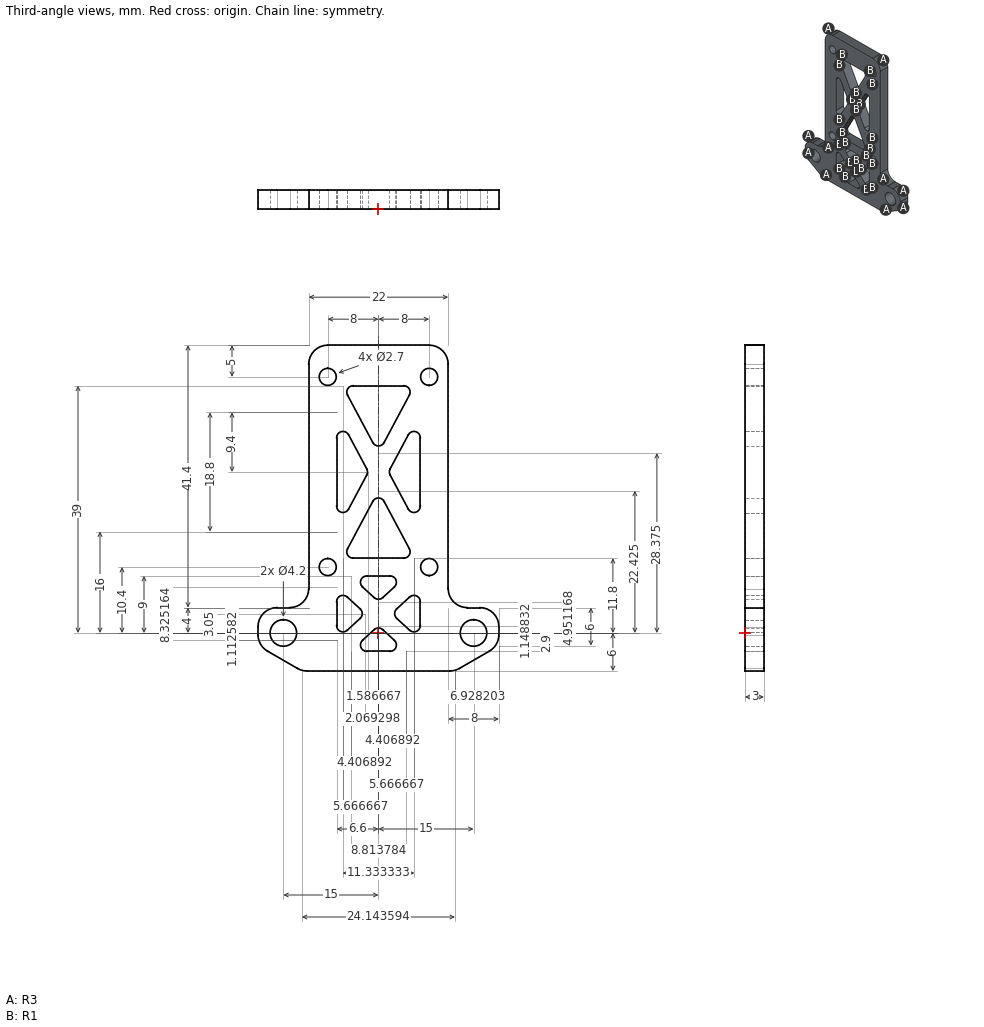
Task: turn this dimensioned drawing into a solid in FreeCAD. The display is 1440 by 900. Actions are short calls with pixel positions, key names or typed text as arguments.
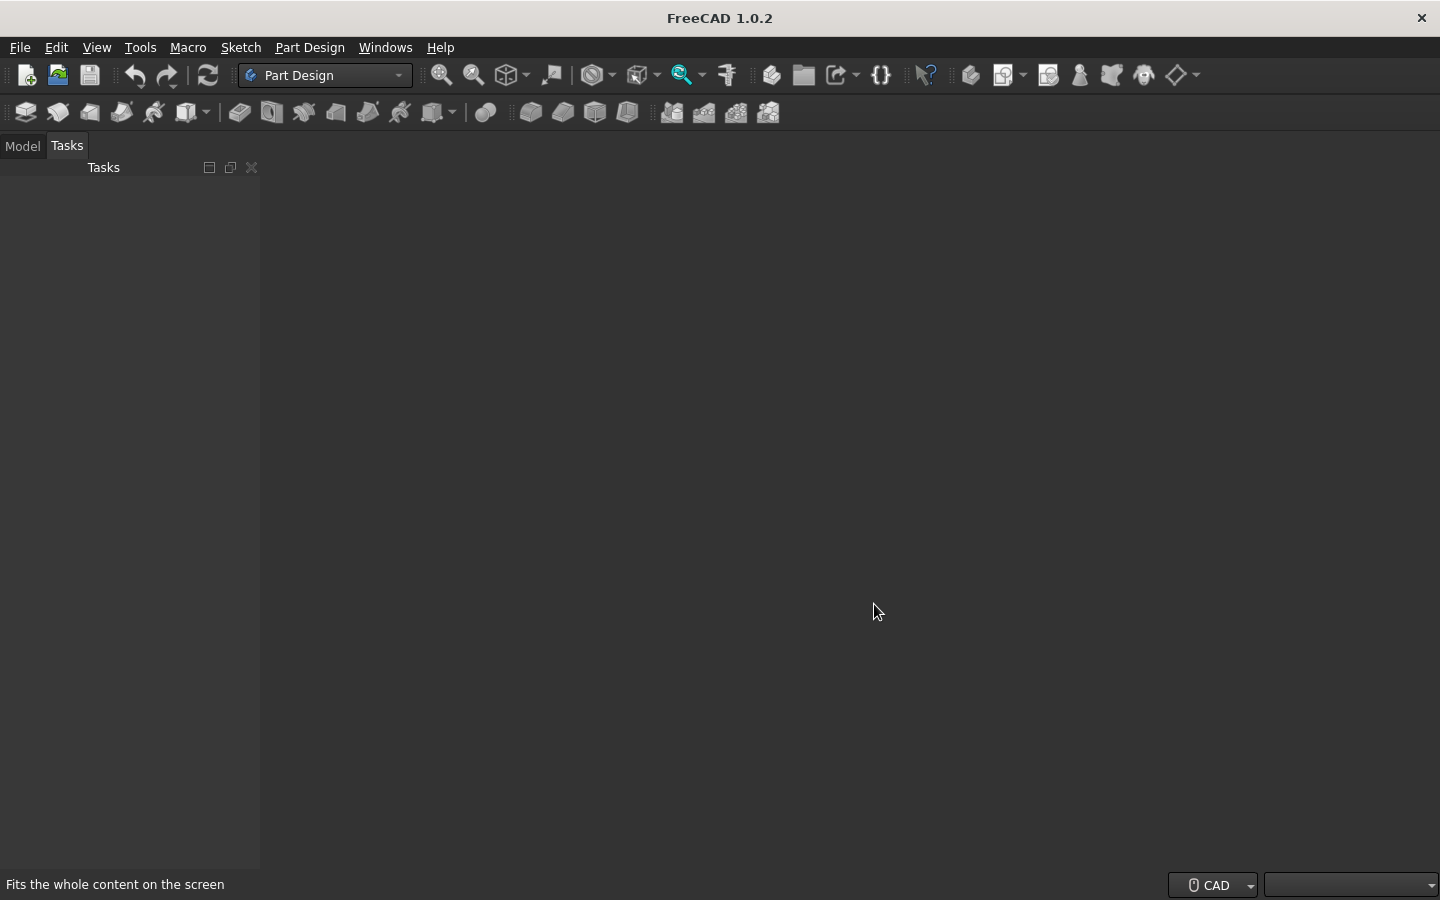
click(26, 76)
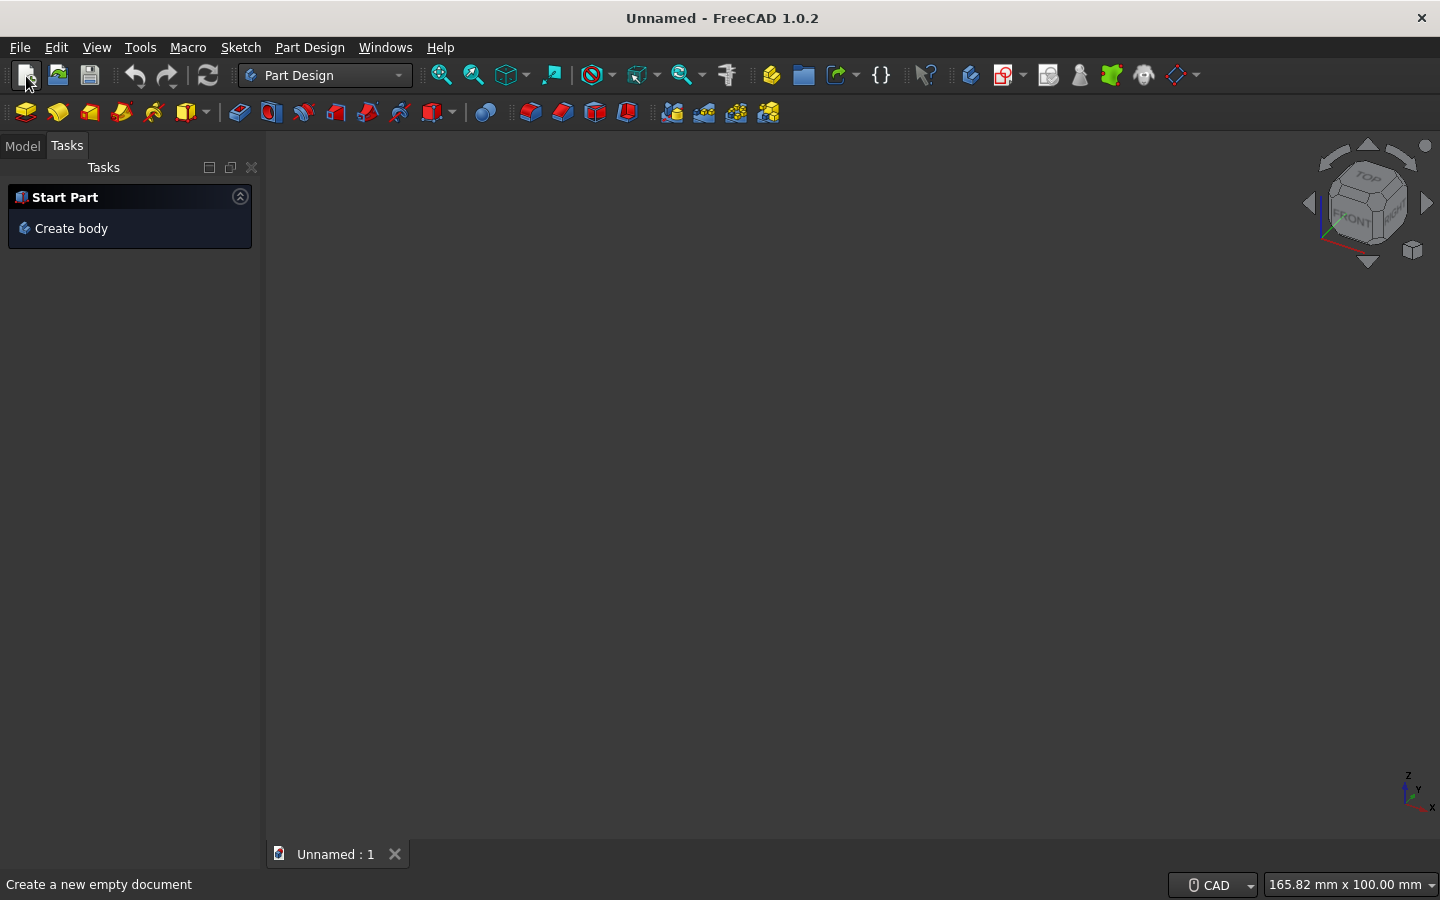
click(1004, 76)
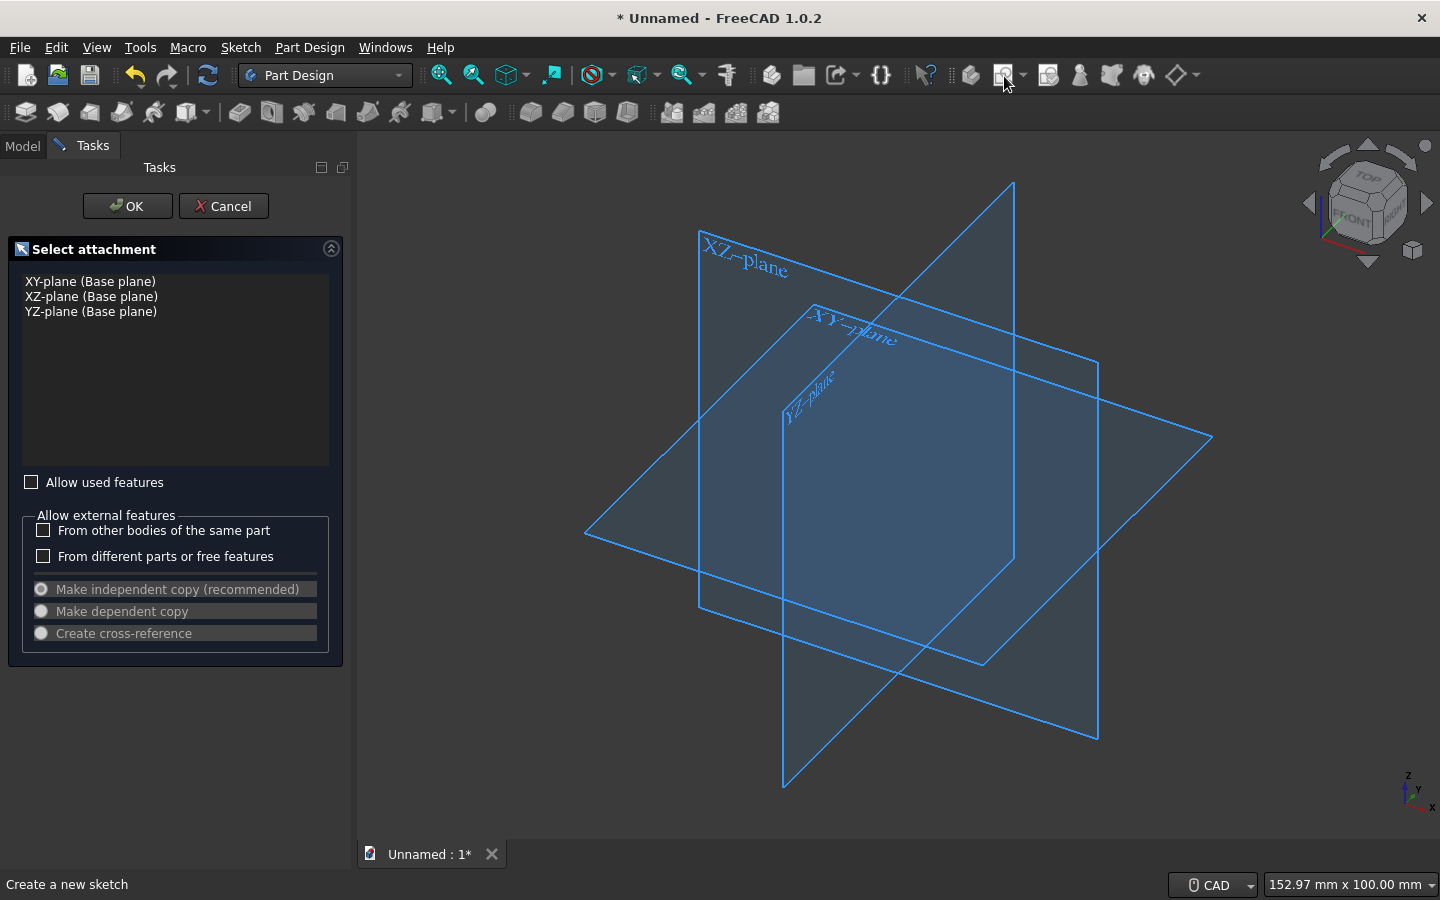
click(82, 296)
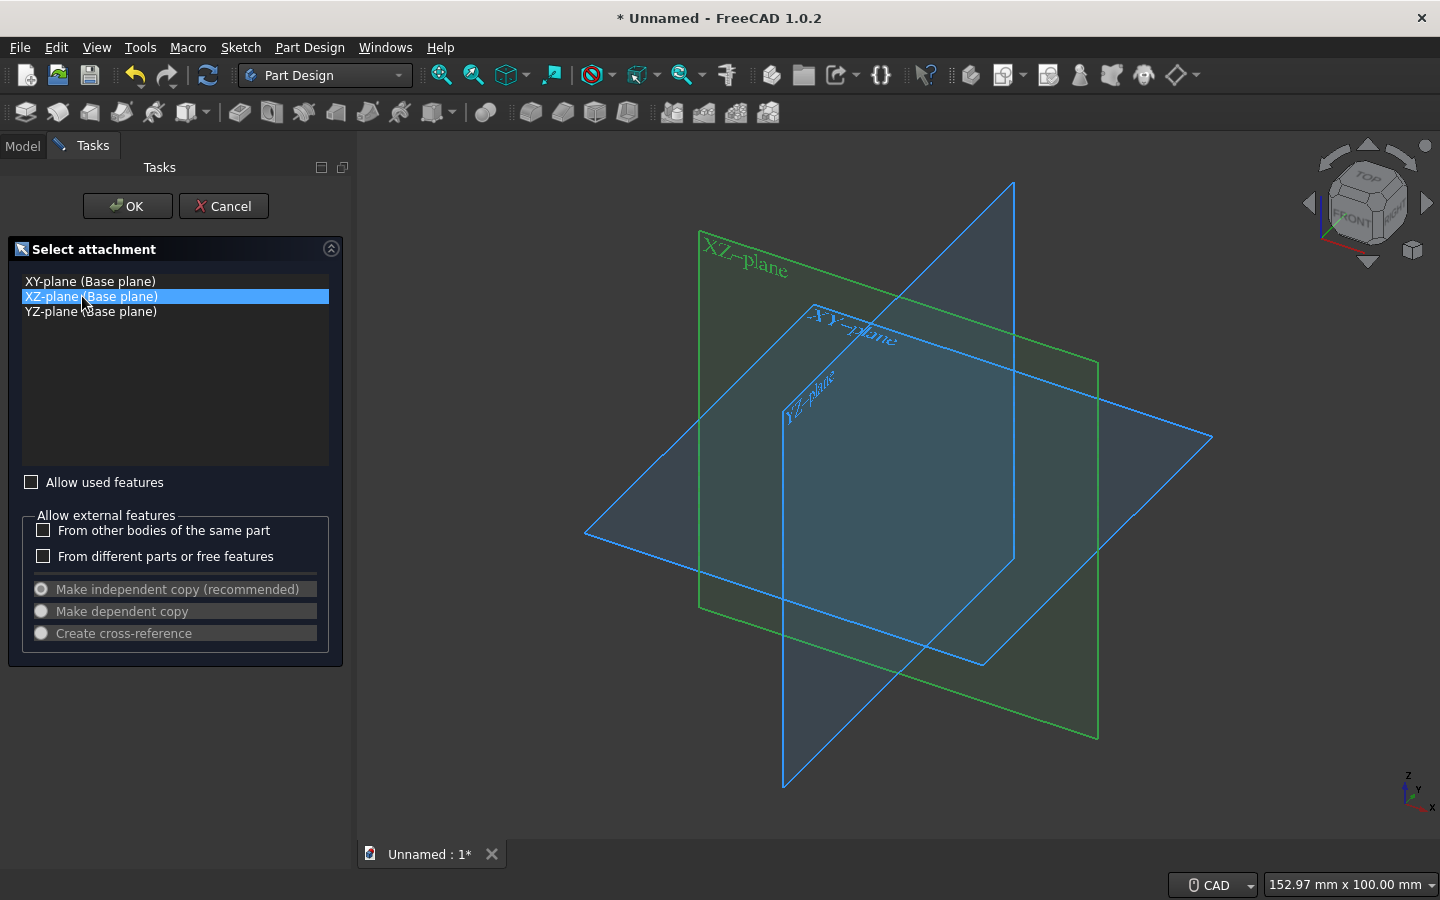
click(128, 206)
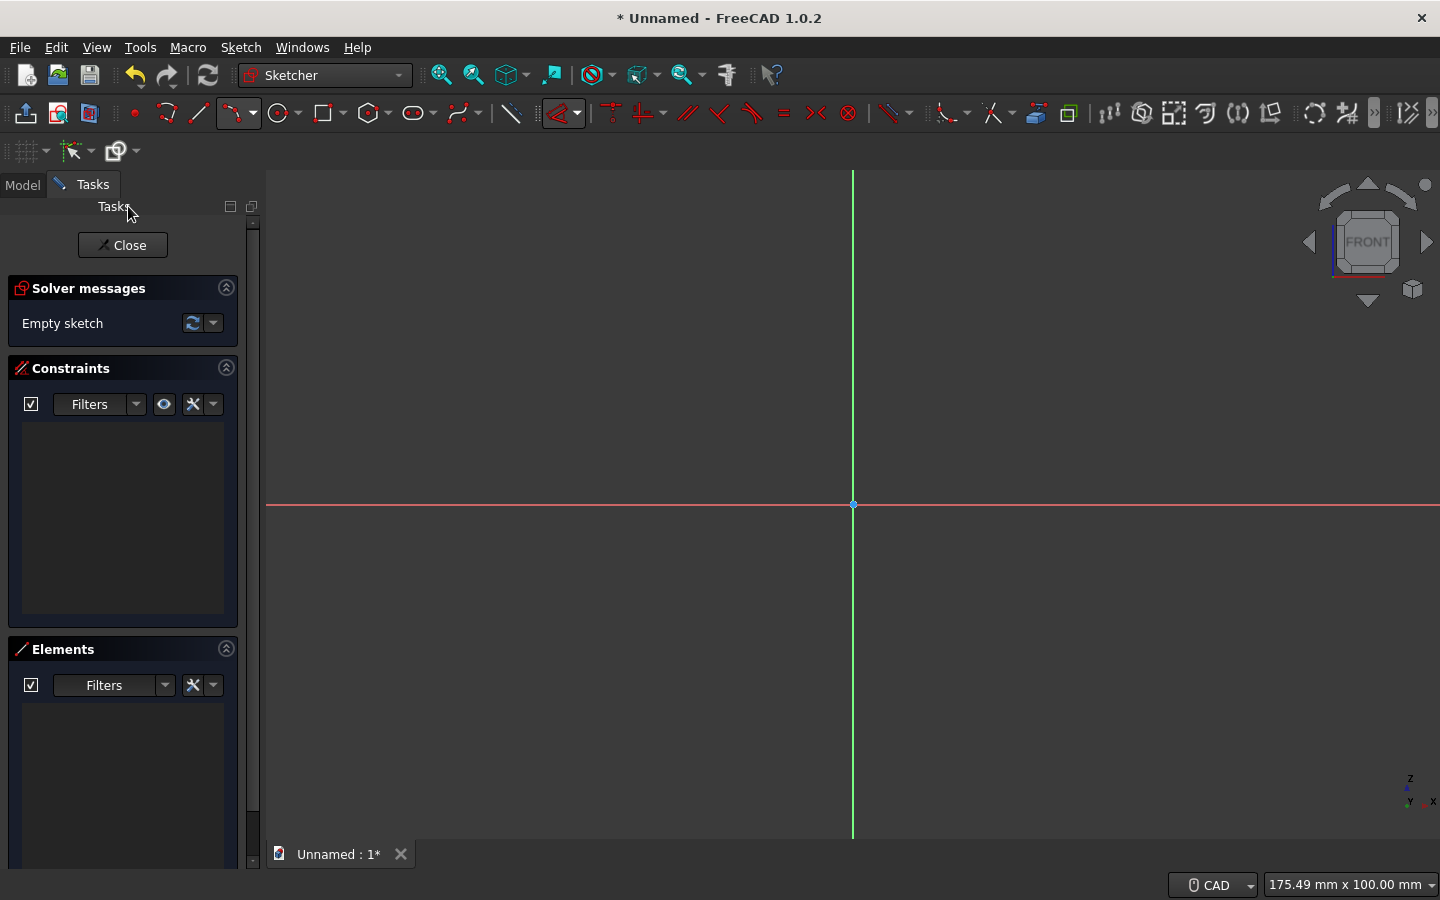
scroll(475, 811, down, 1)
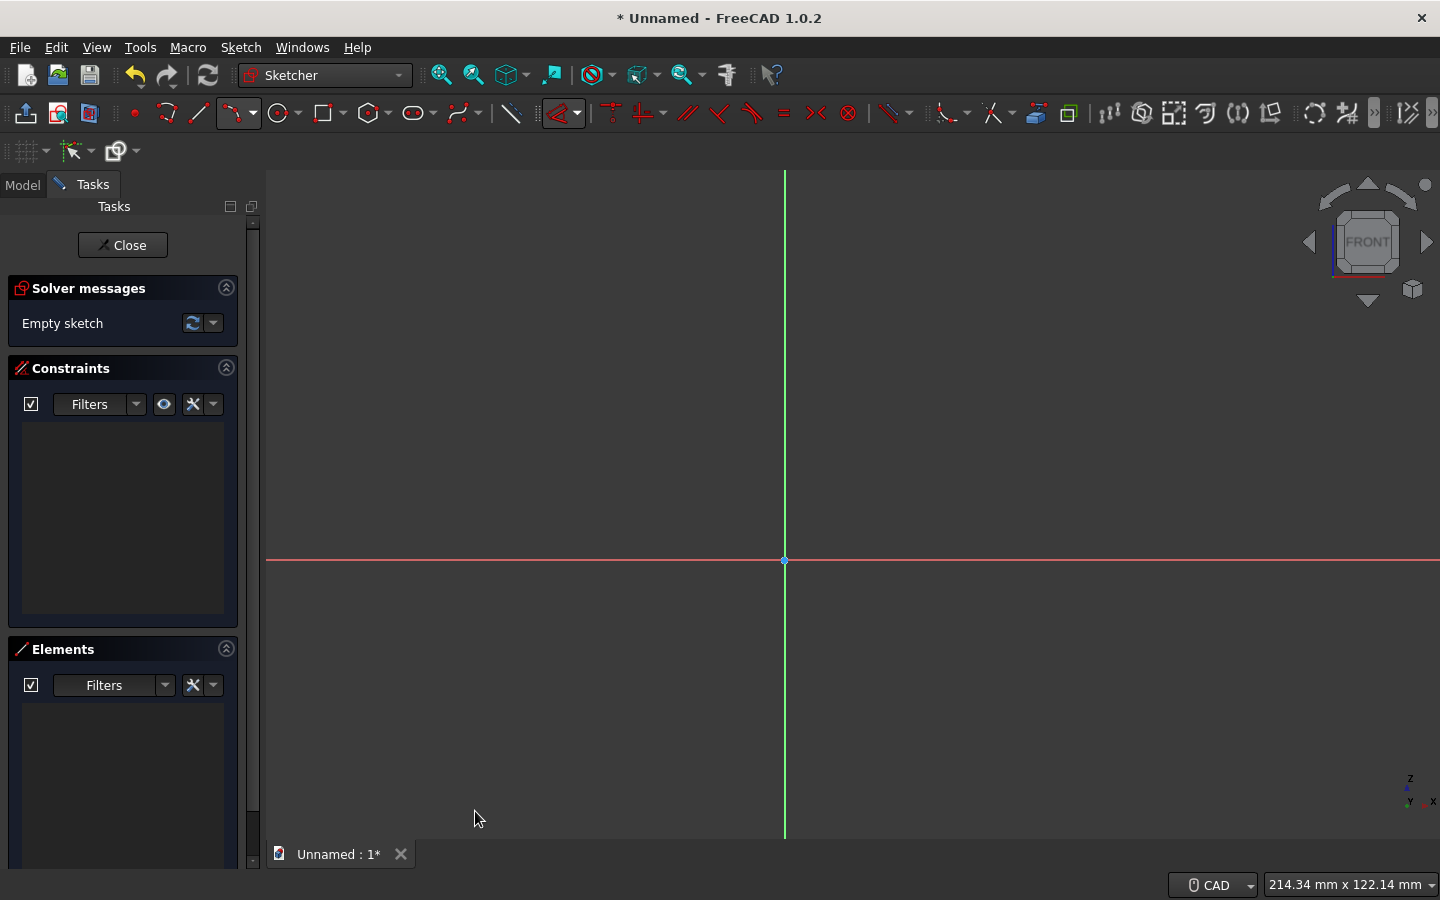
scroll(785, 346, up, 2)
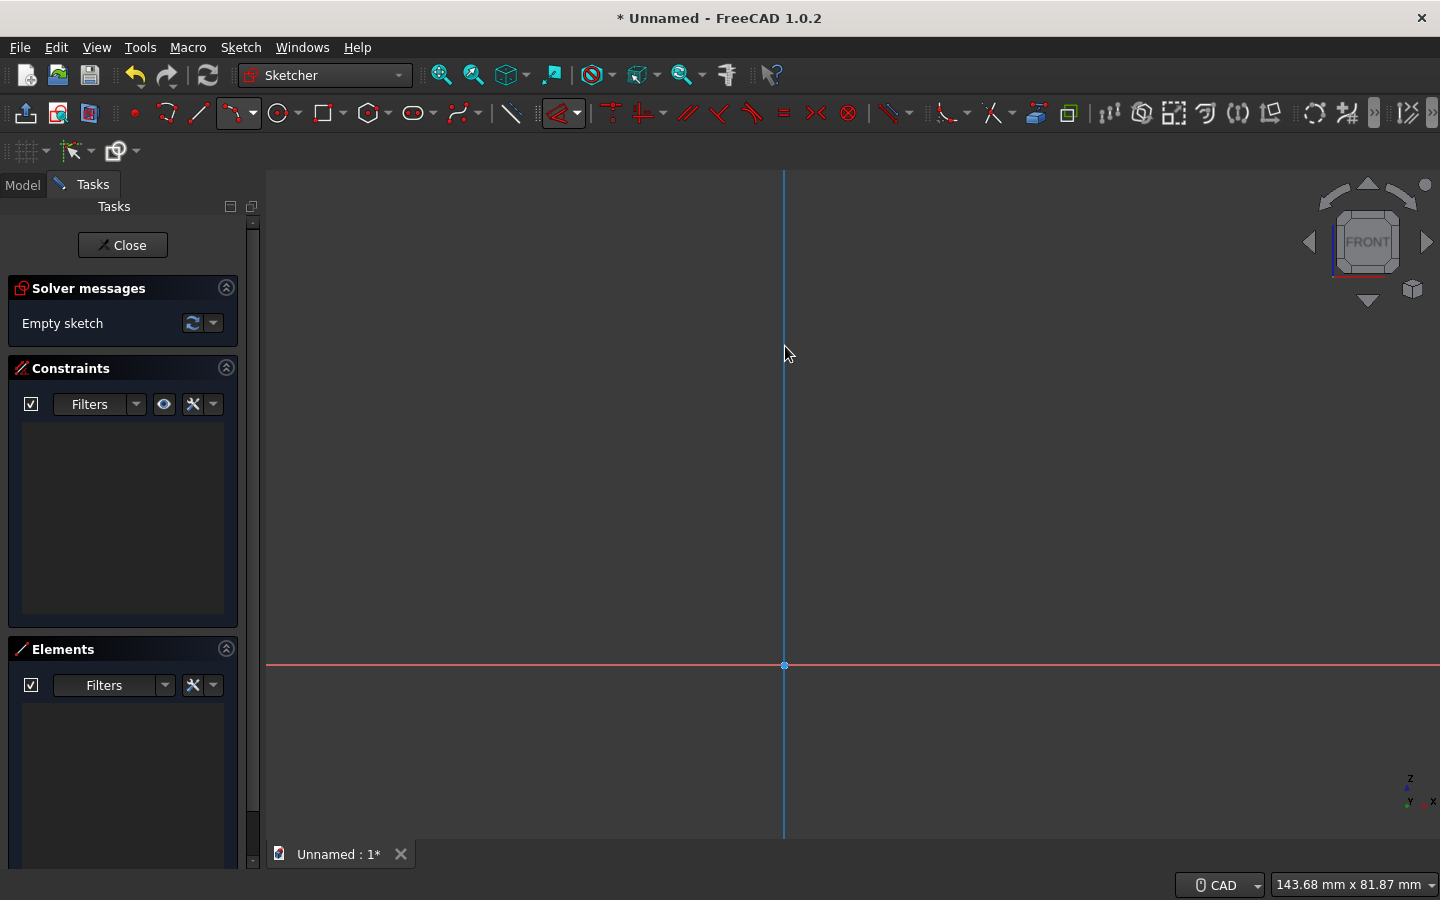
key(g)
key(m)